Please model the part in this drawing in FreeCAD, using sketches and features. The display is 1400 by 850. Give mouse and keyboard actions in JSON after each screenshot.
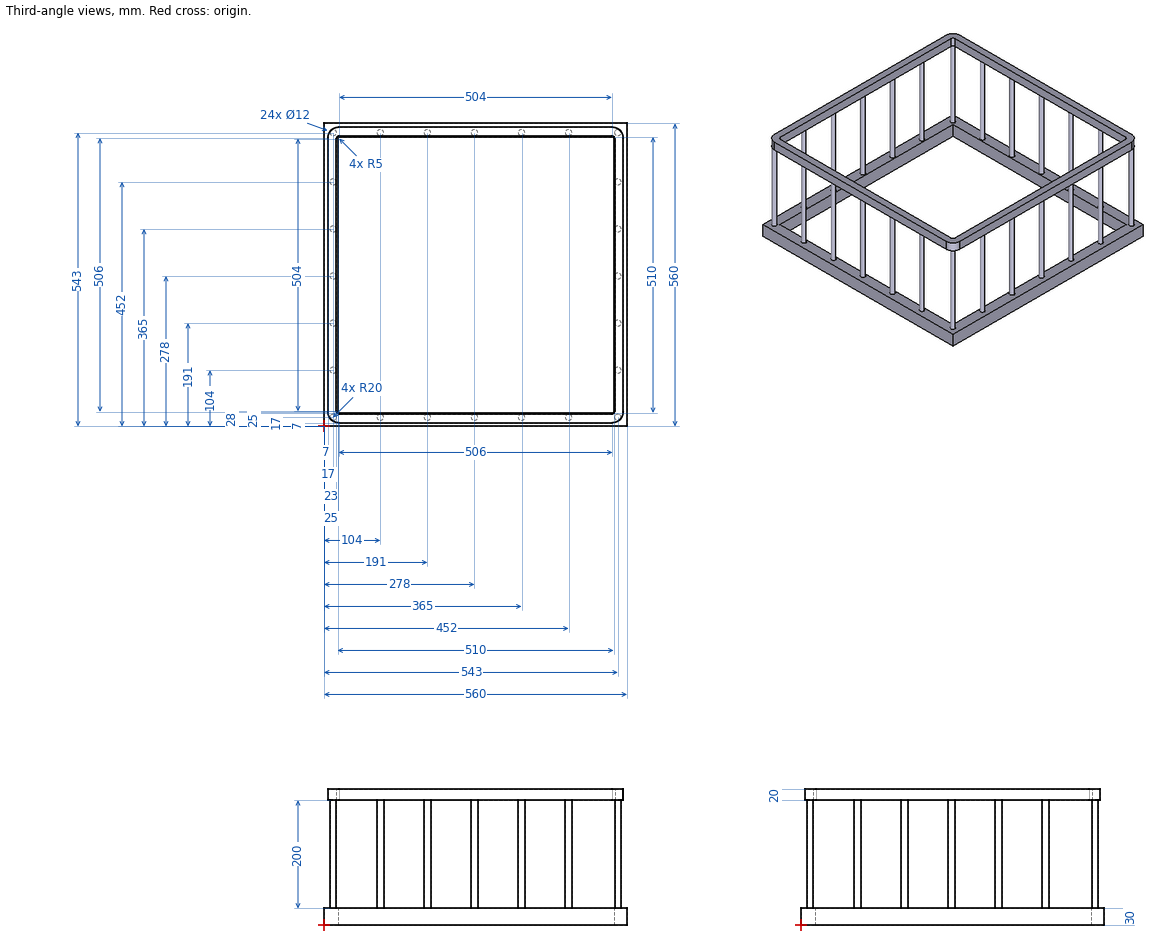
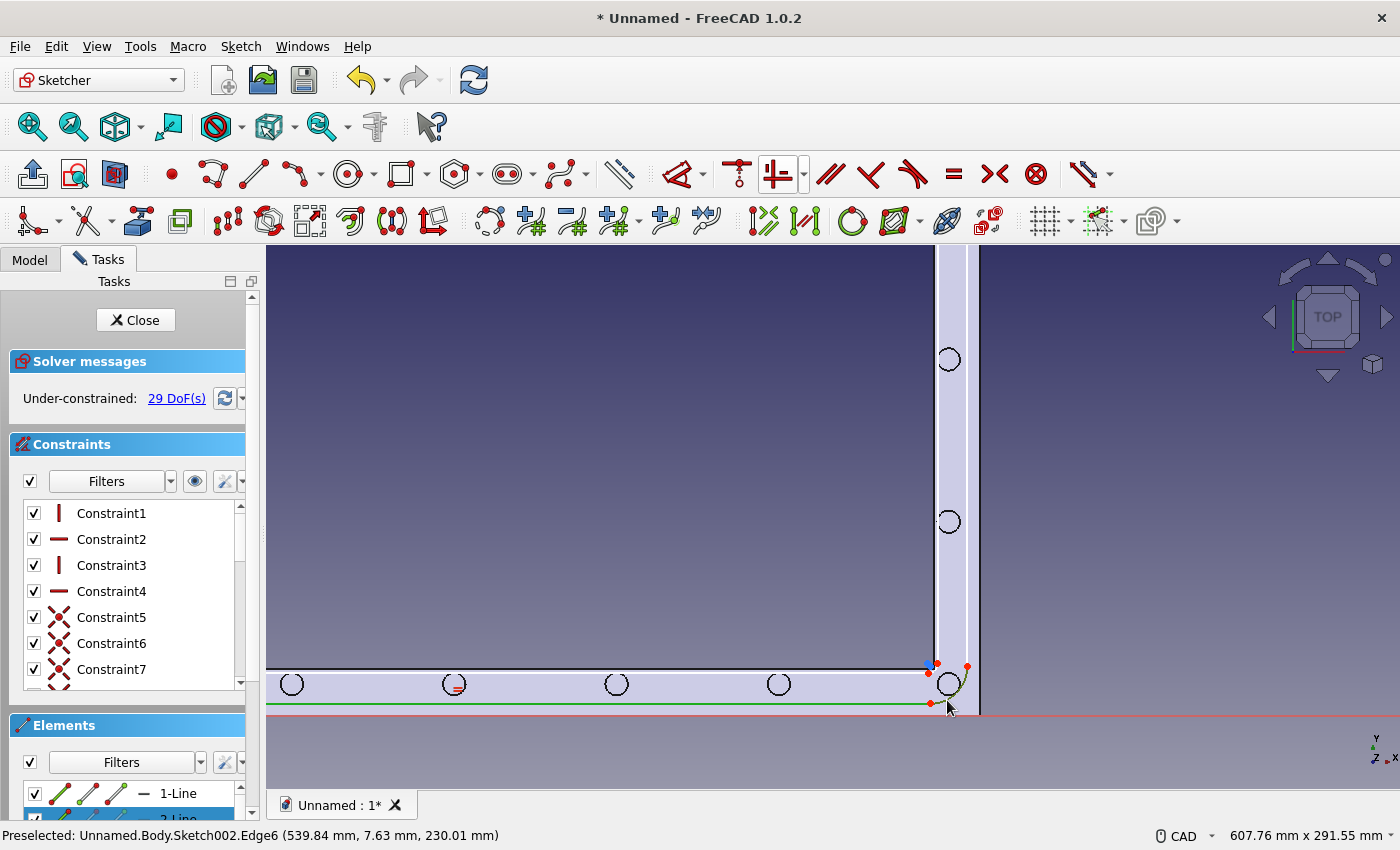
{"action": "left_click", "coordinate": [913, 174]}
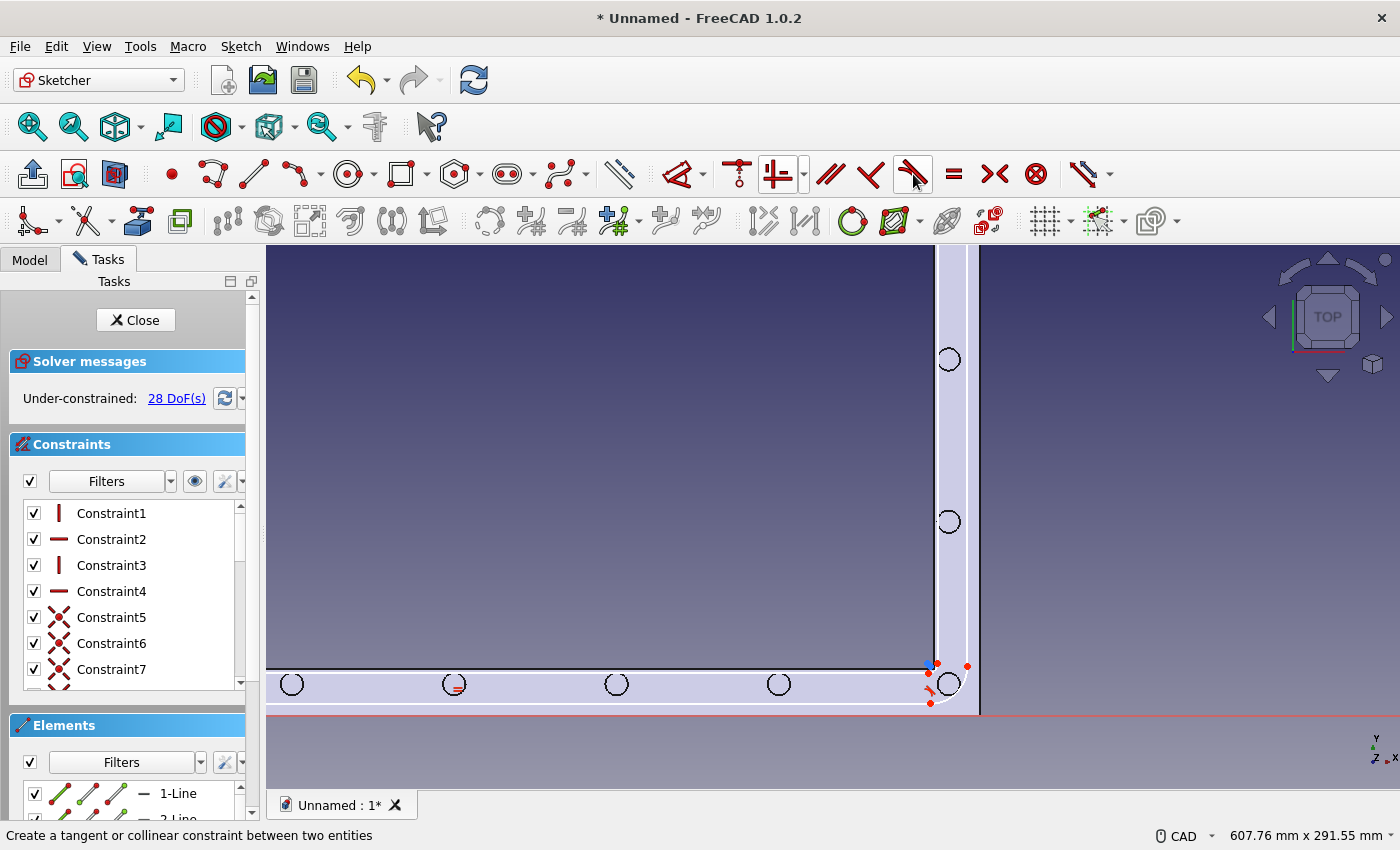
{"action": "left_click", "coordinate": [967, 384]}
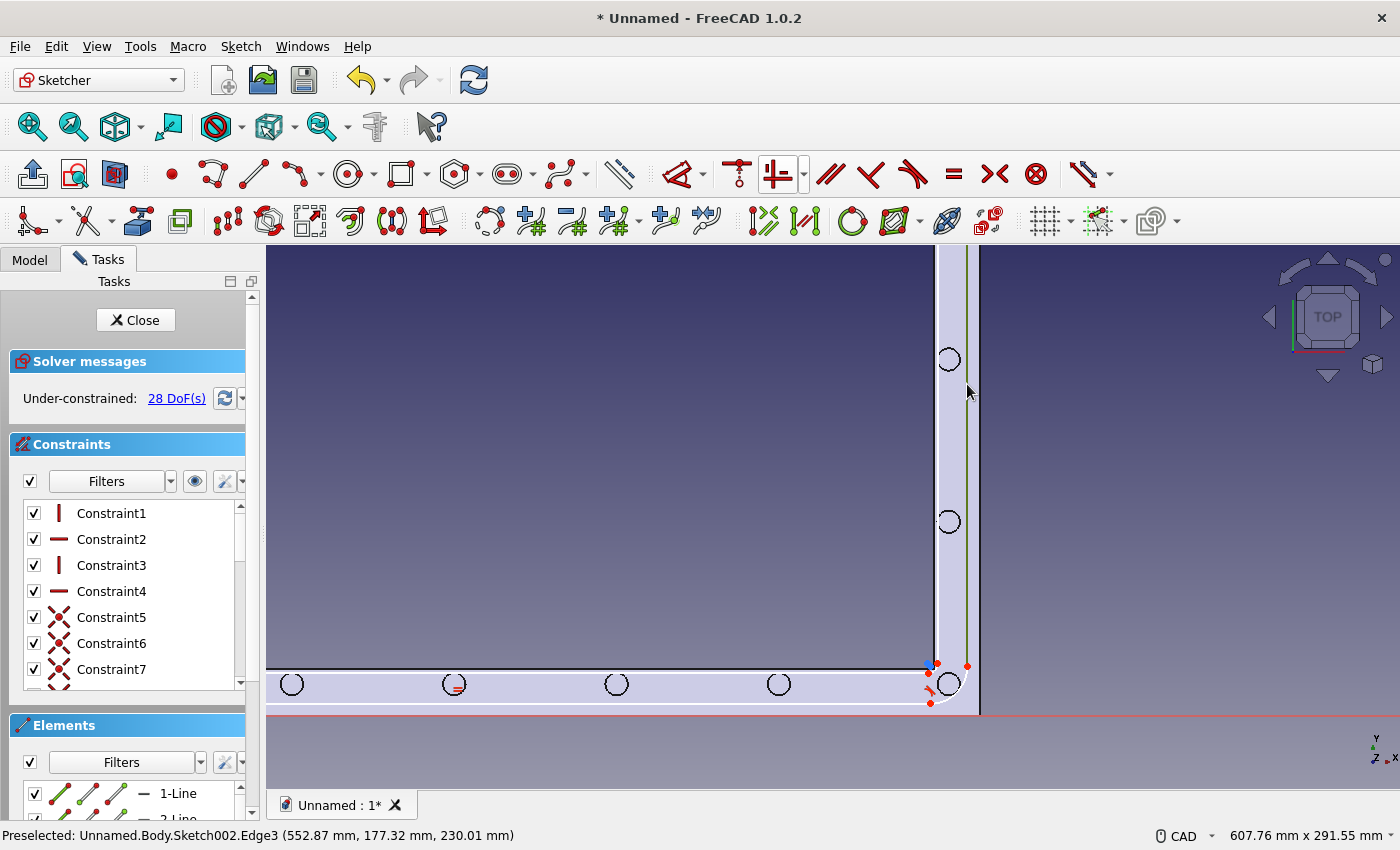
{"action": "left_click", "coordinate": [947, 700]}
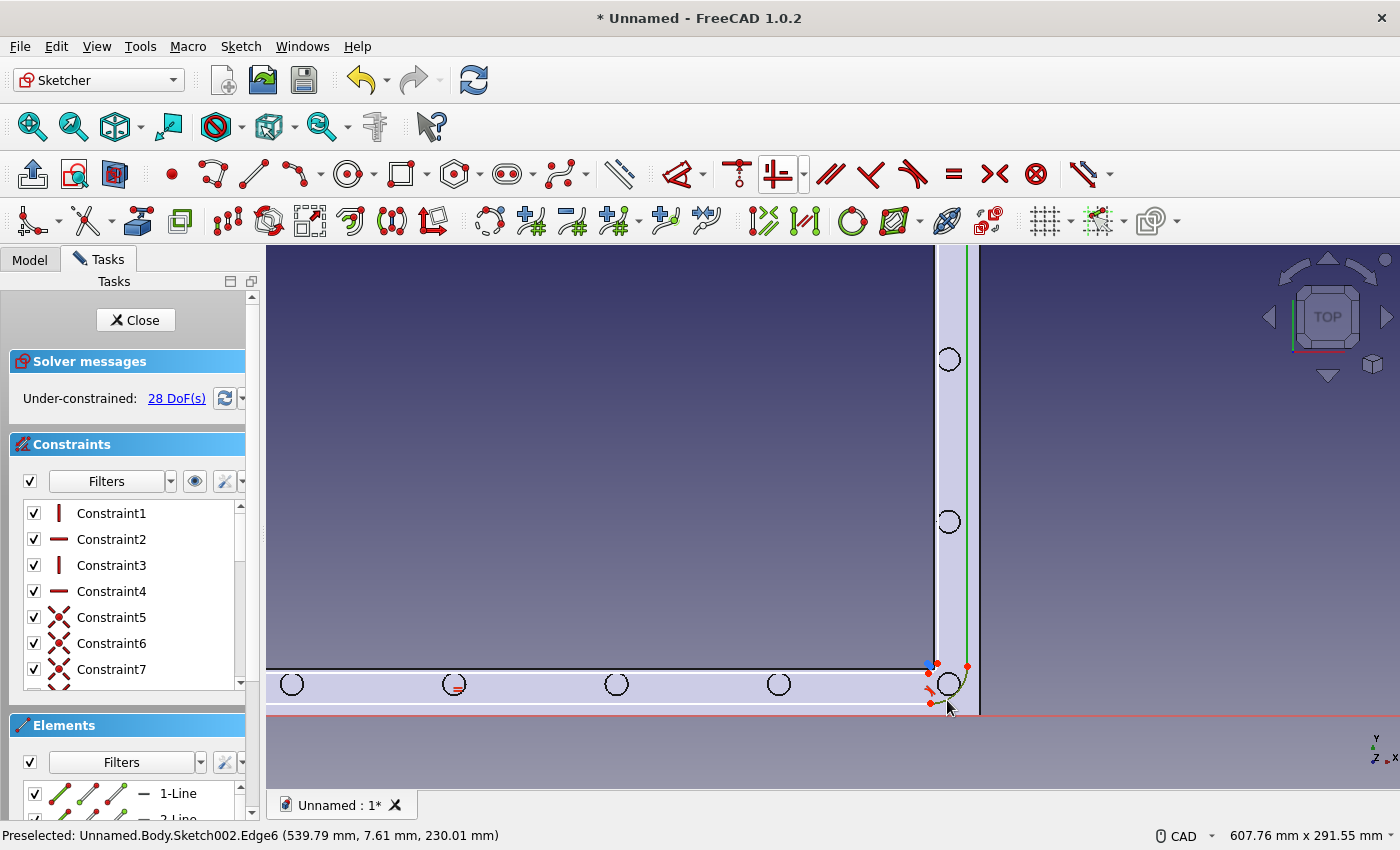
{"action": "left_click", "coordinate": [913, 174]}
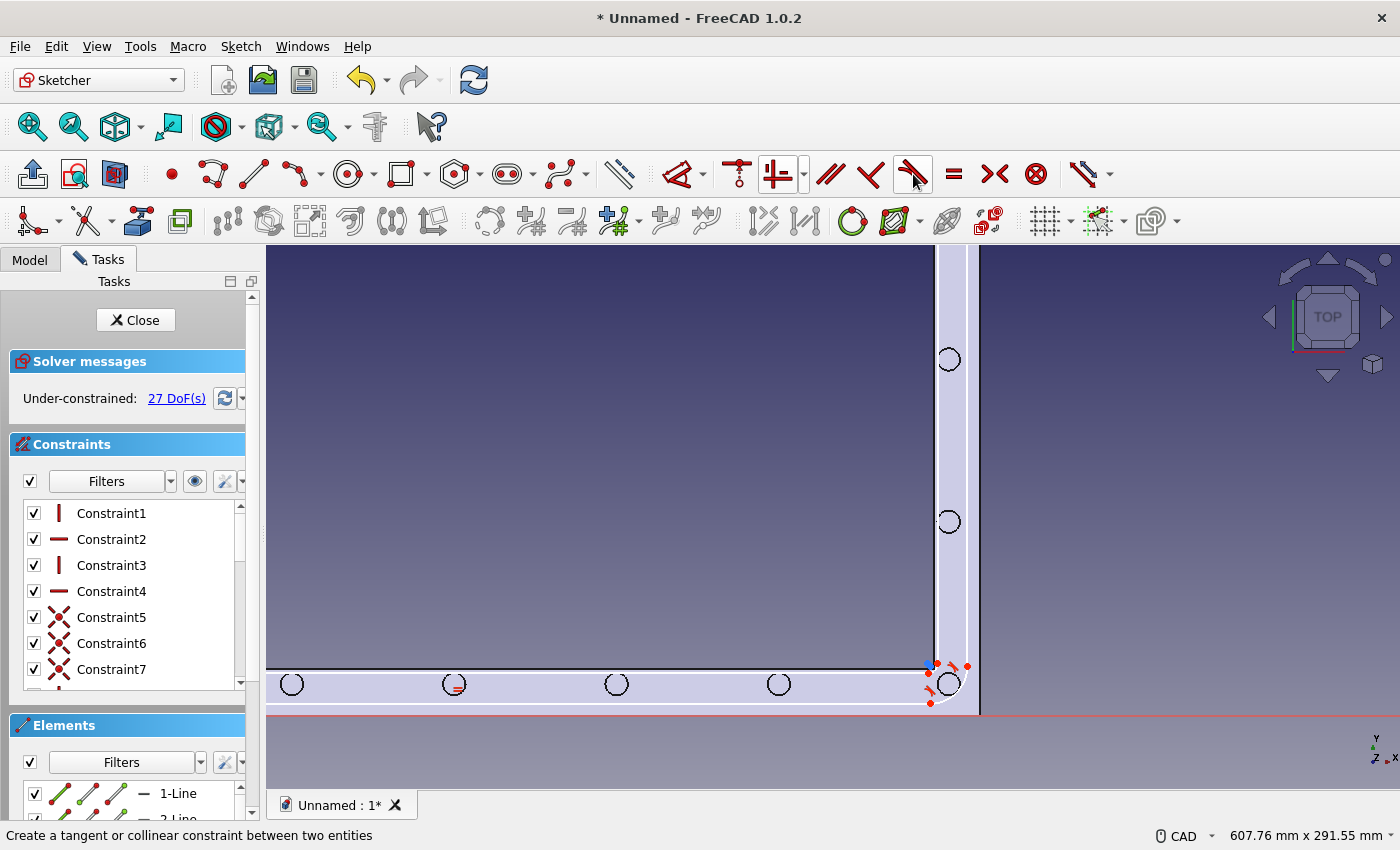
{"action": "left_click", "coordinate": [967, 384]}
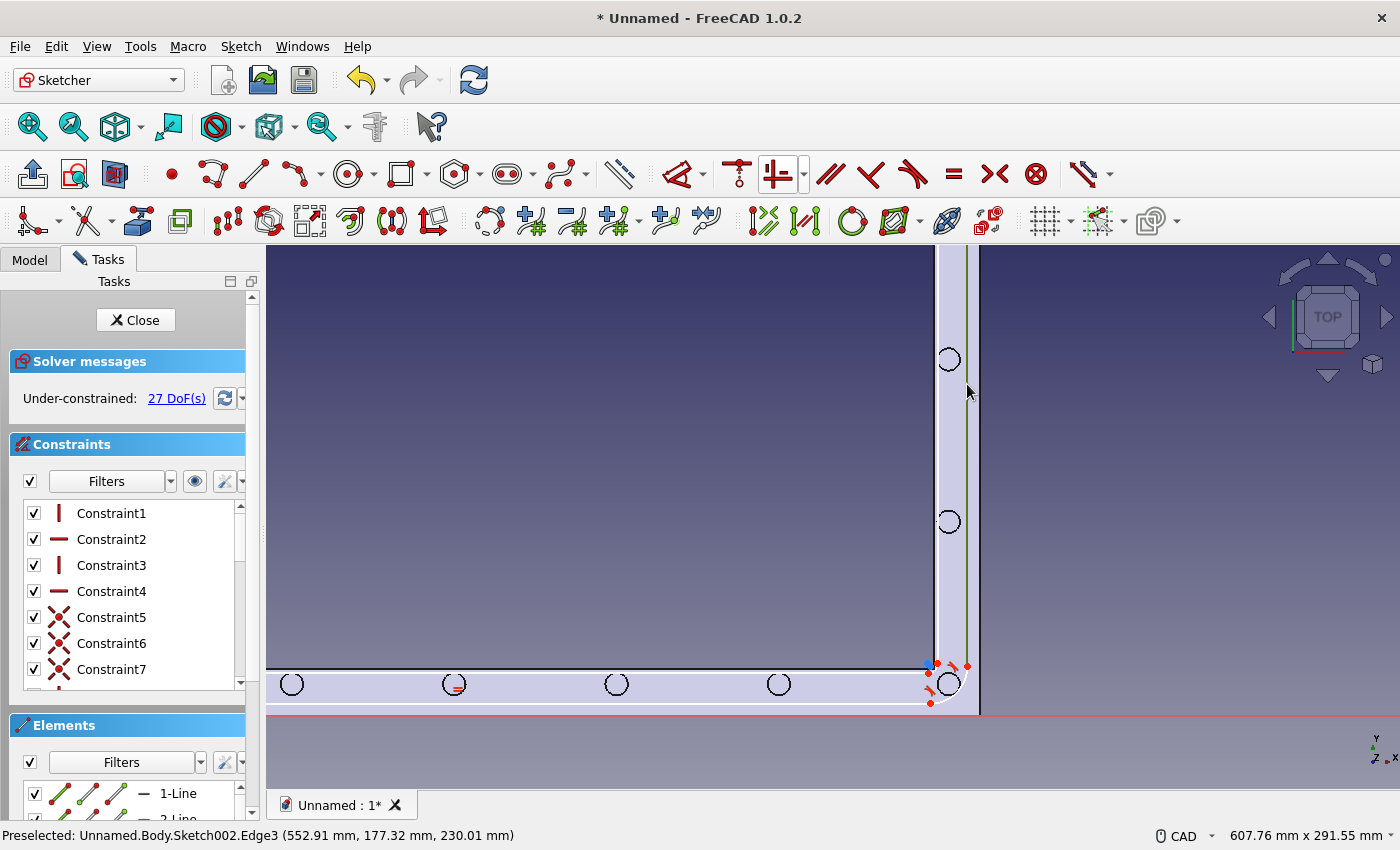
{"action": "scroll", "coordinate": [947, 702], "scroll_direction": "down", "scroll_amount": 5}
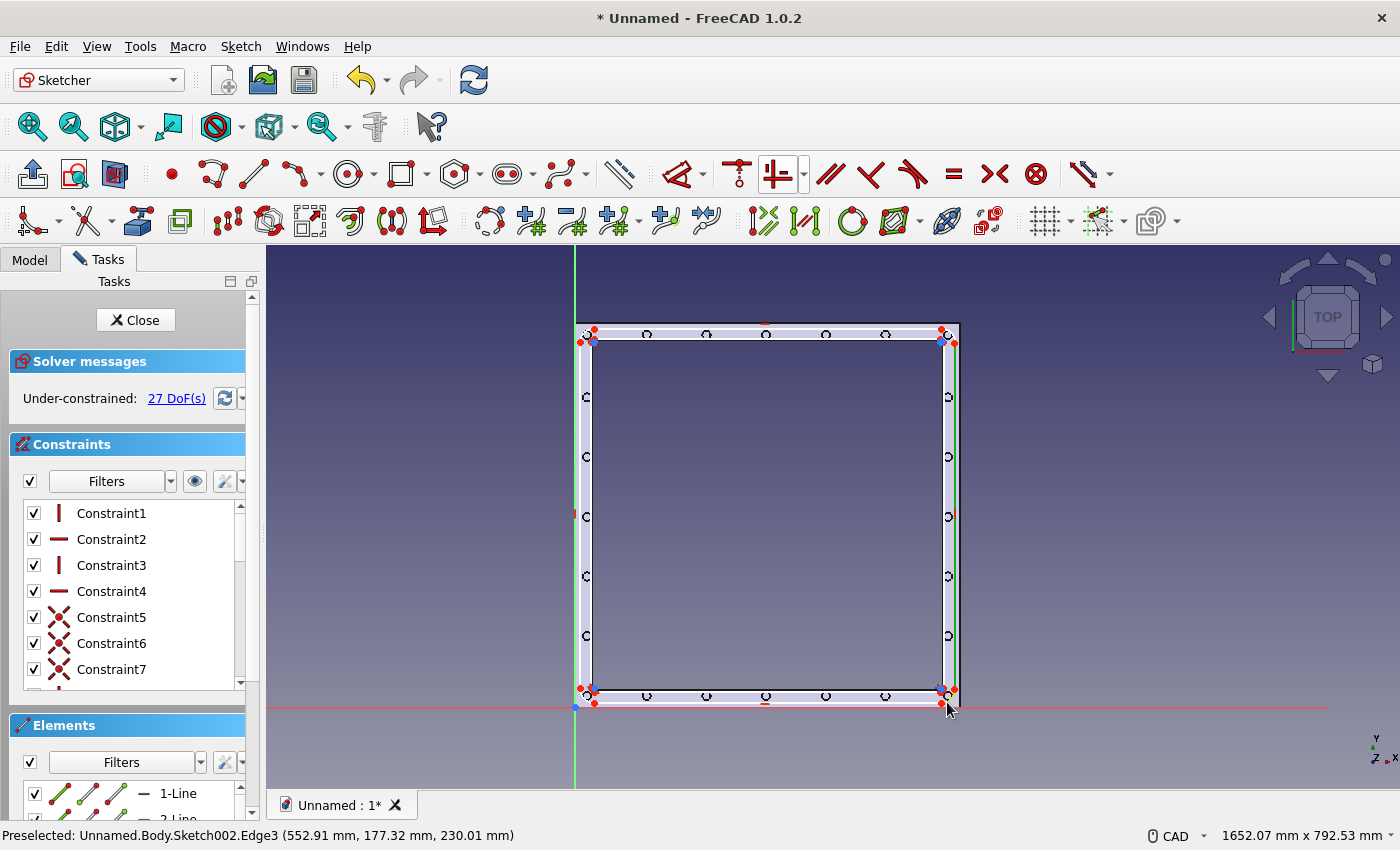
{"action": "scroll", "coordinate": [954, 336], "scroll_direction": "up", "scroll_amount": 4}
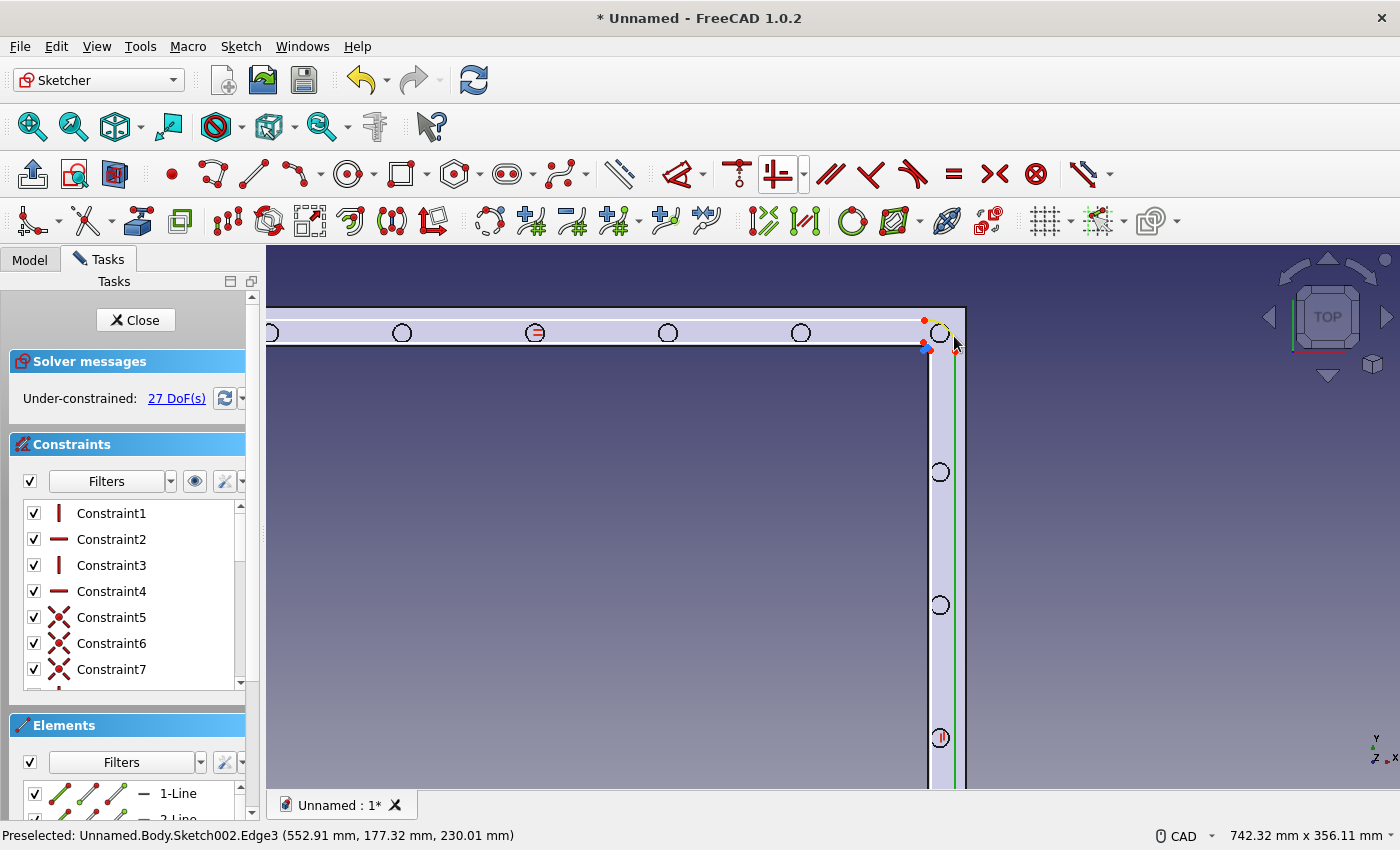
{"action": "left_click", "coordinate": [953, 337]}